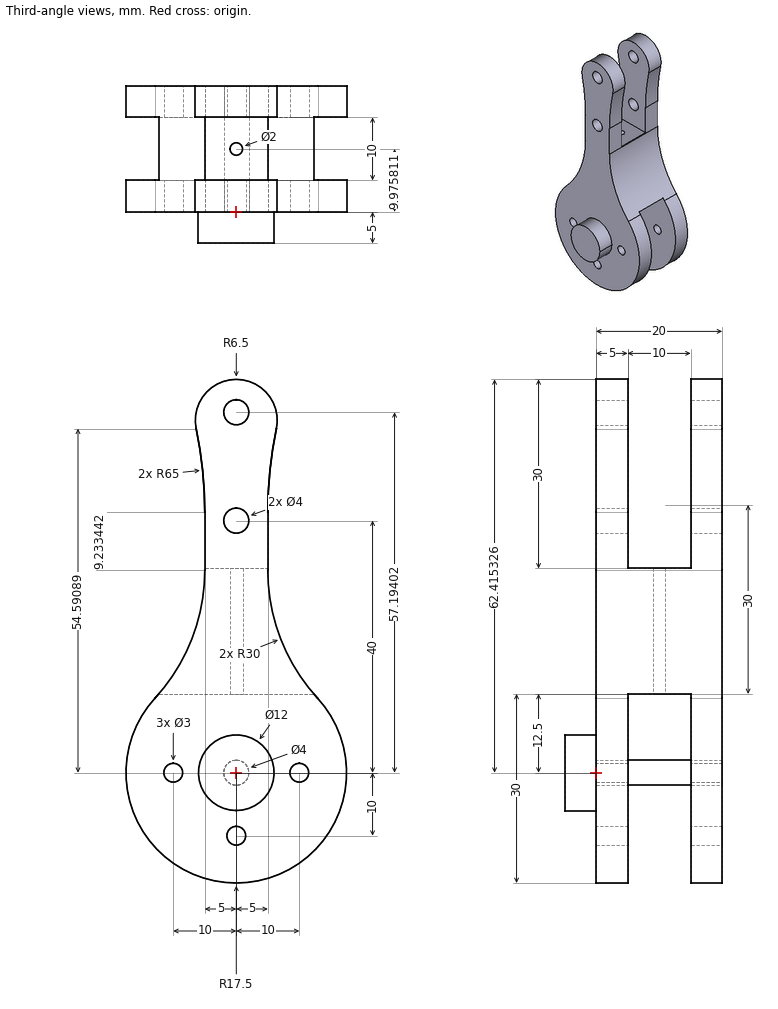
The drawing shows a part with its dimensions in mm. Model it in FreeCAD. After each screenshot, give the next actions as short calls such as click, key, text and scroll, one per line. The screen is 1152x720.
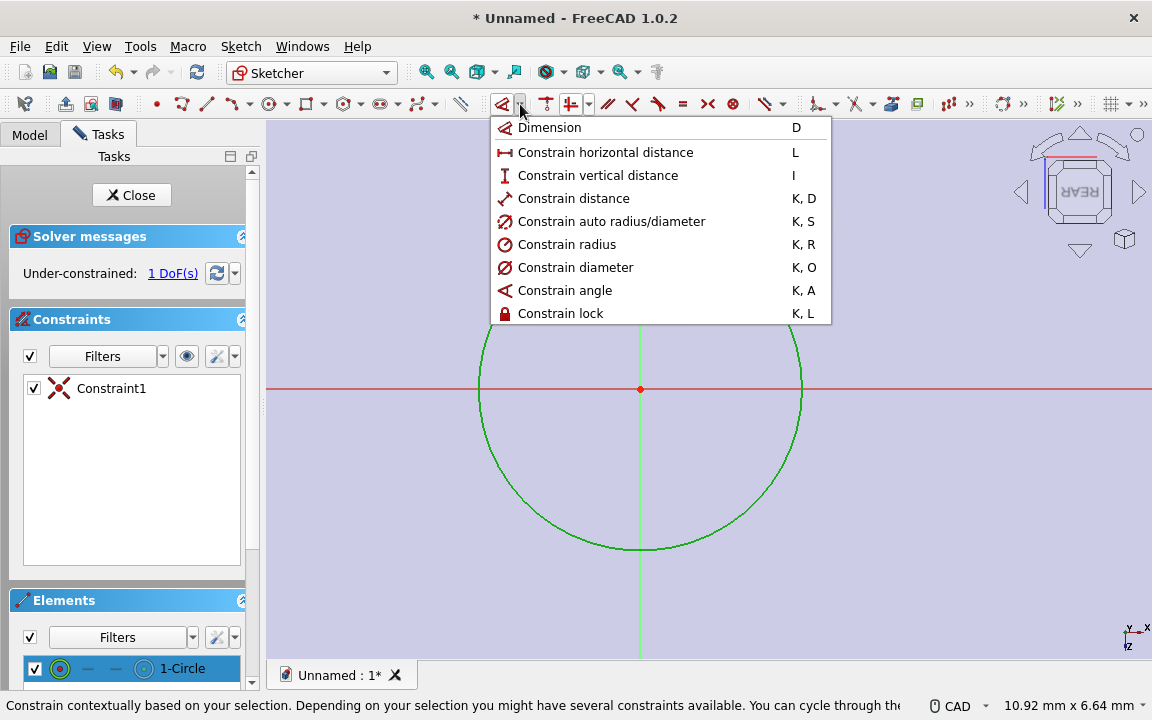
click(661, 268)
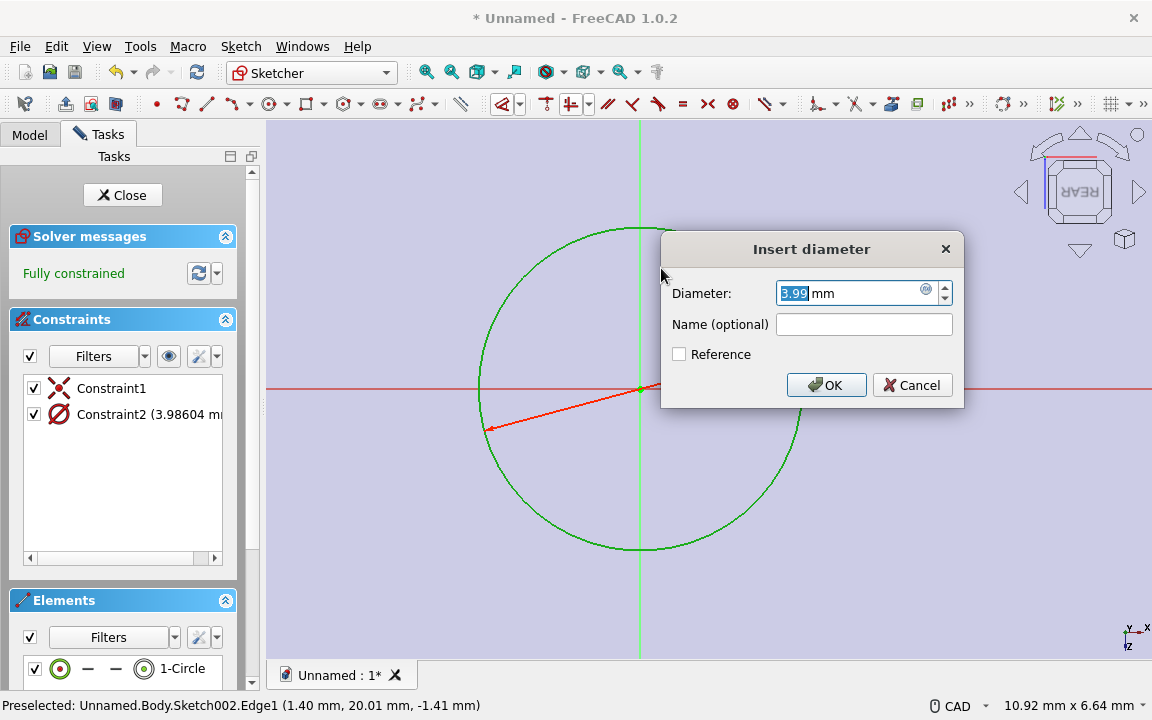
text(4)
key(Return)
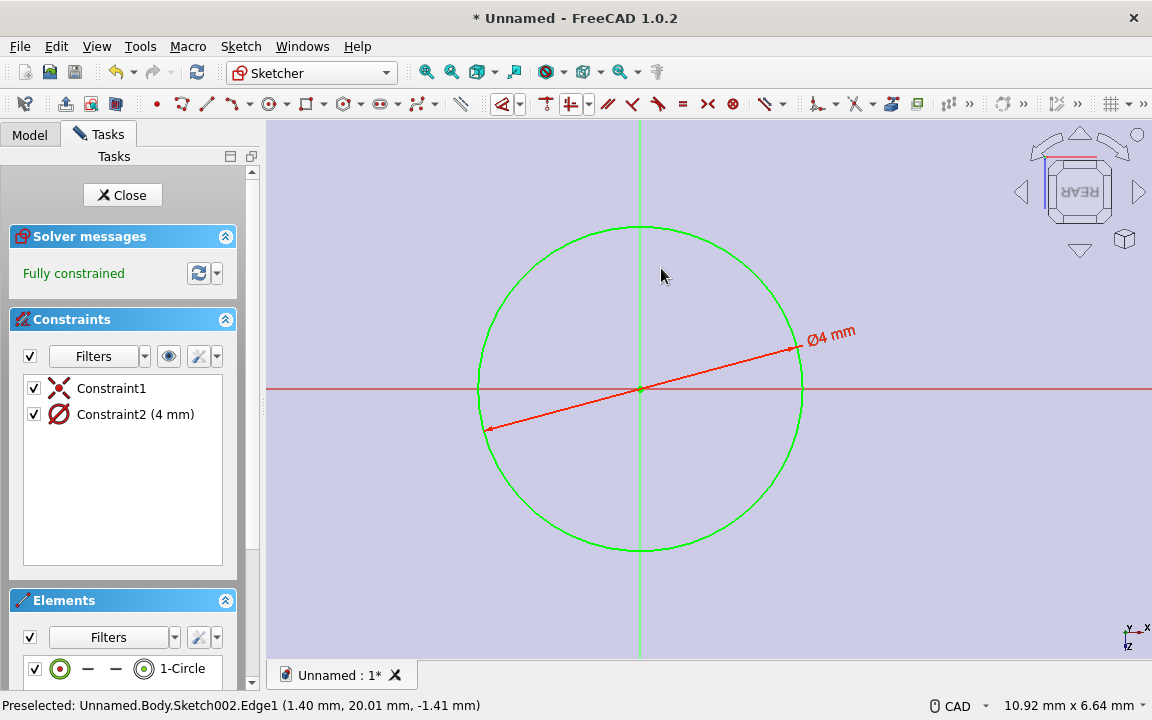
click(123, 195)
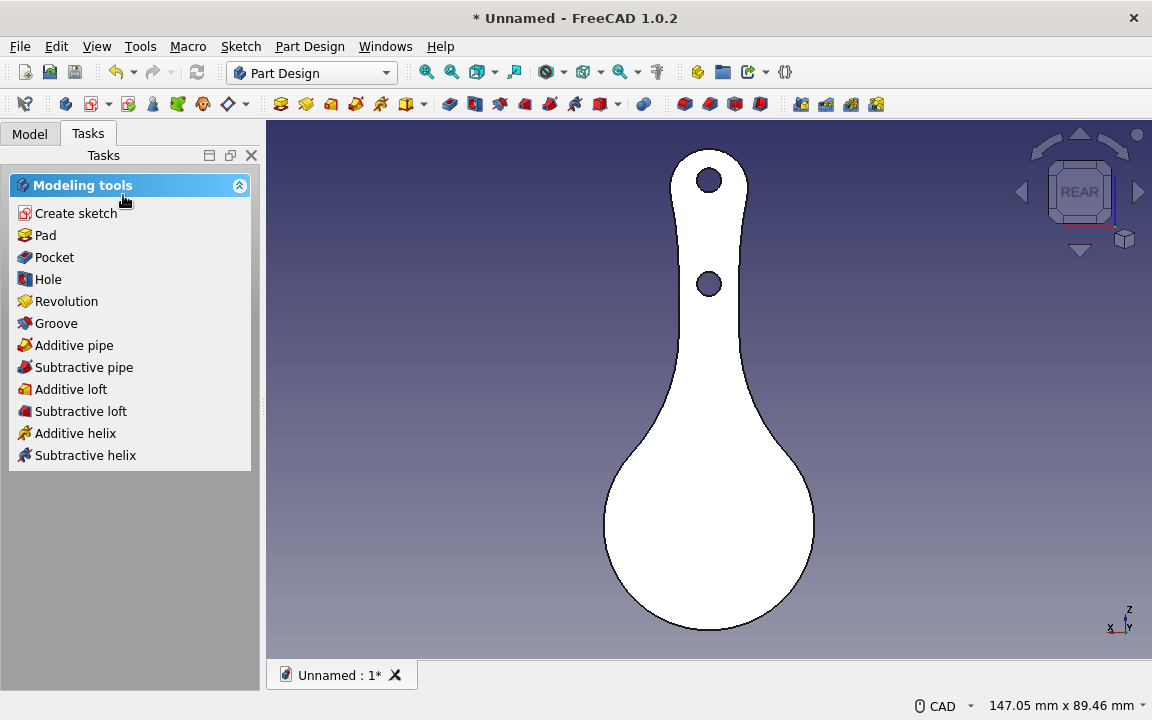
click(450, 104)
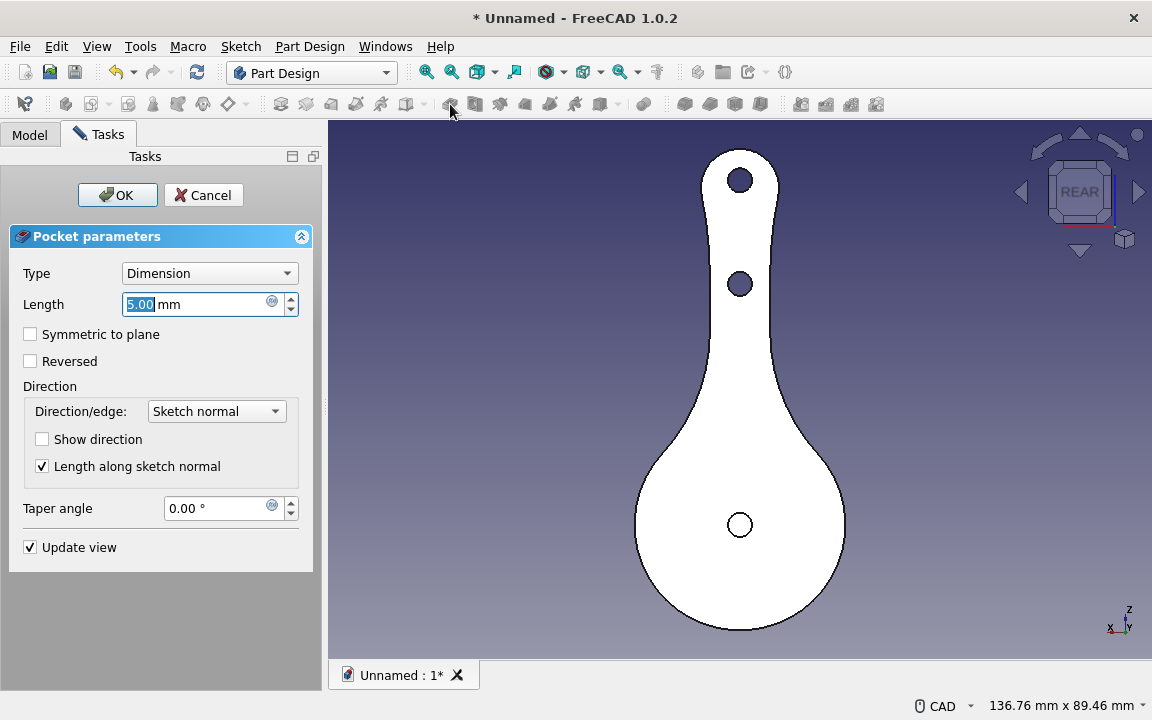
click(210, 274)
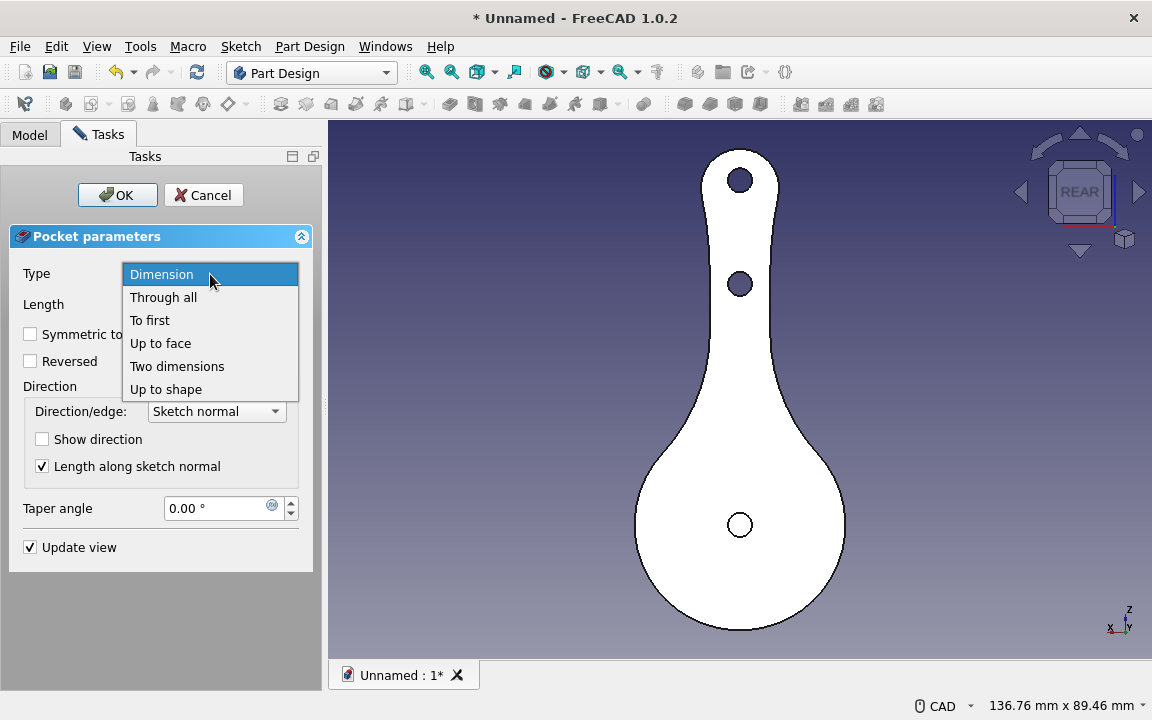
click(208, 298)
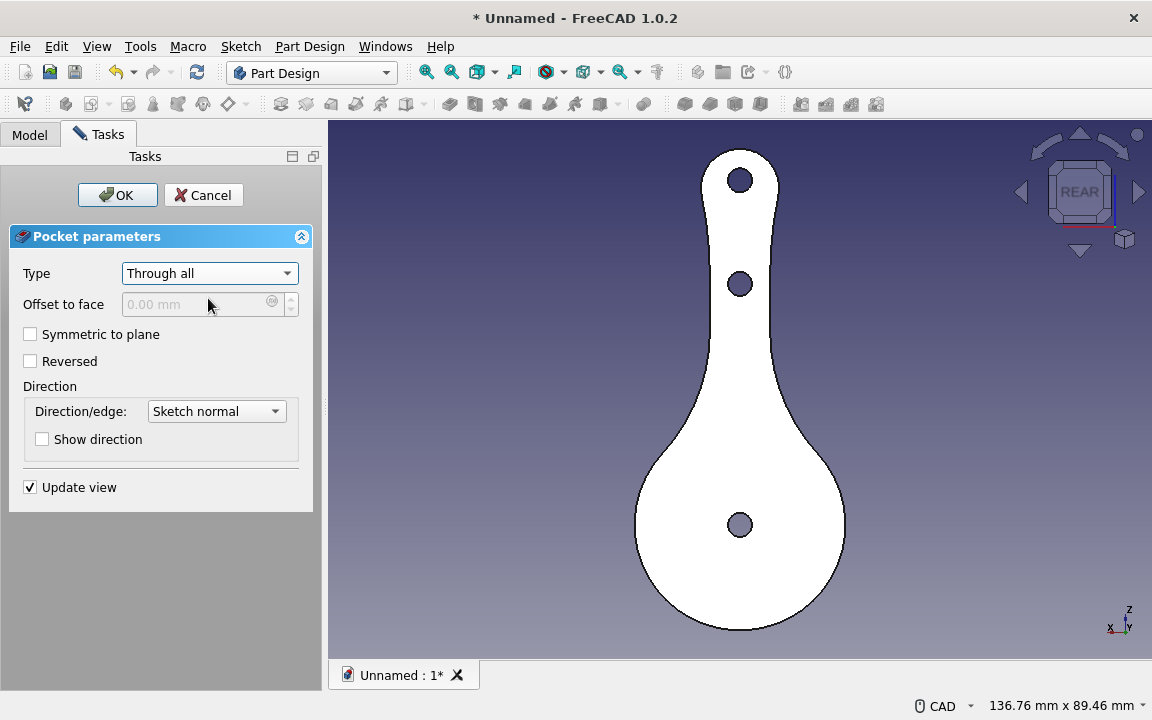
click(118, 195)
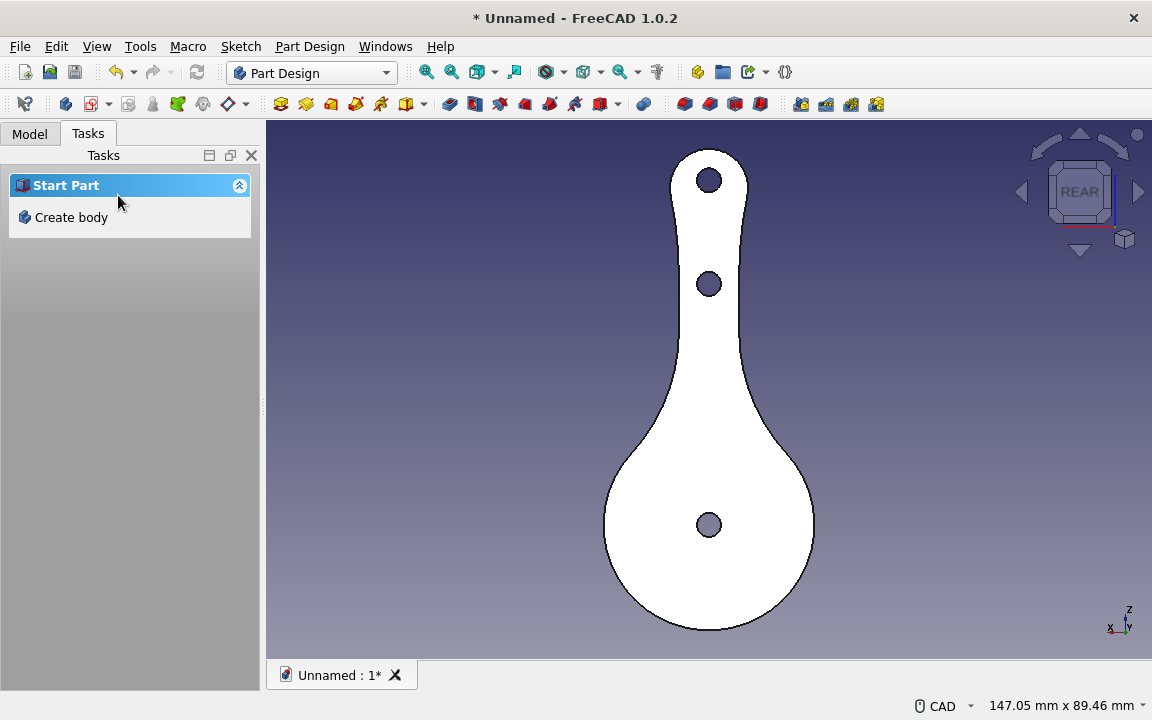
click(709, 457)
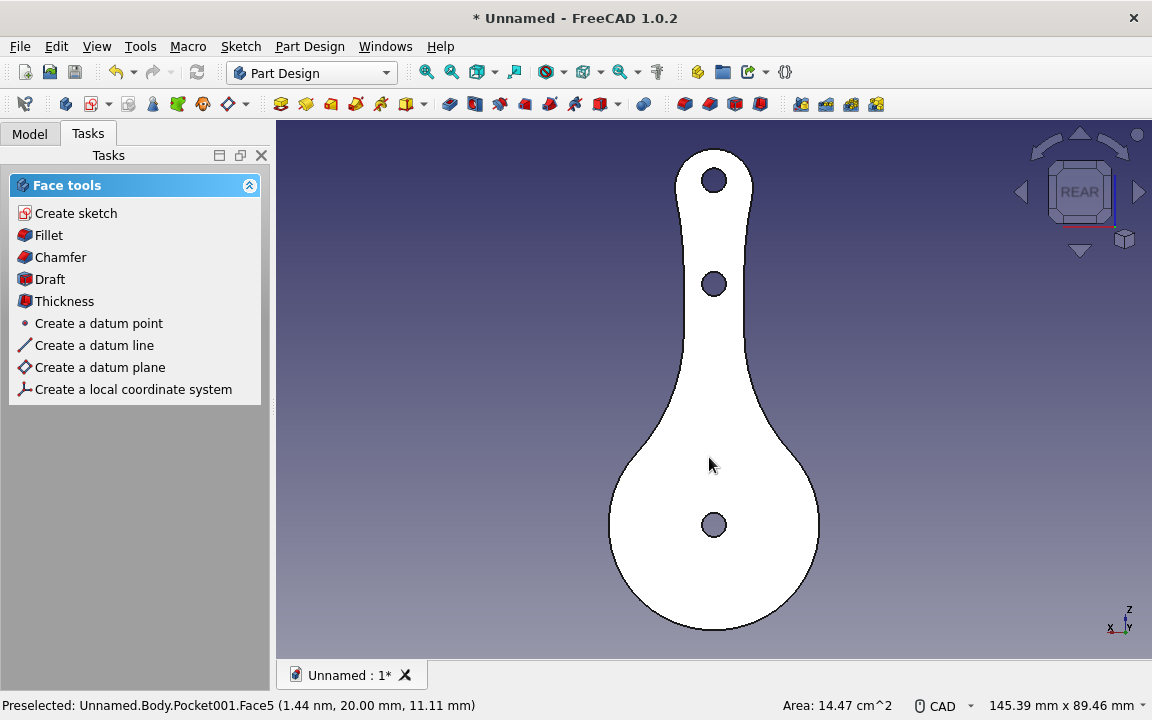
click(90, 104)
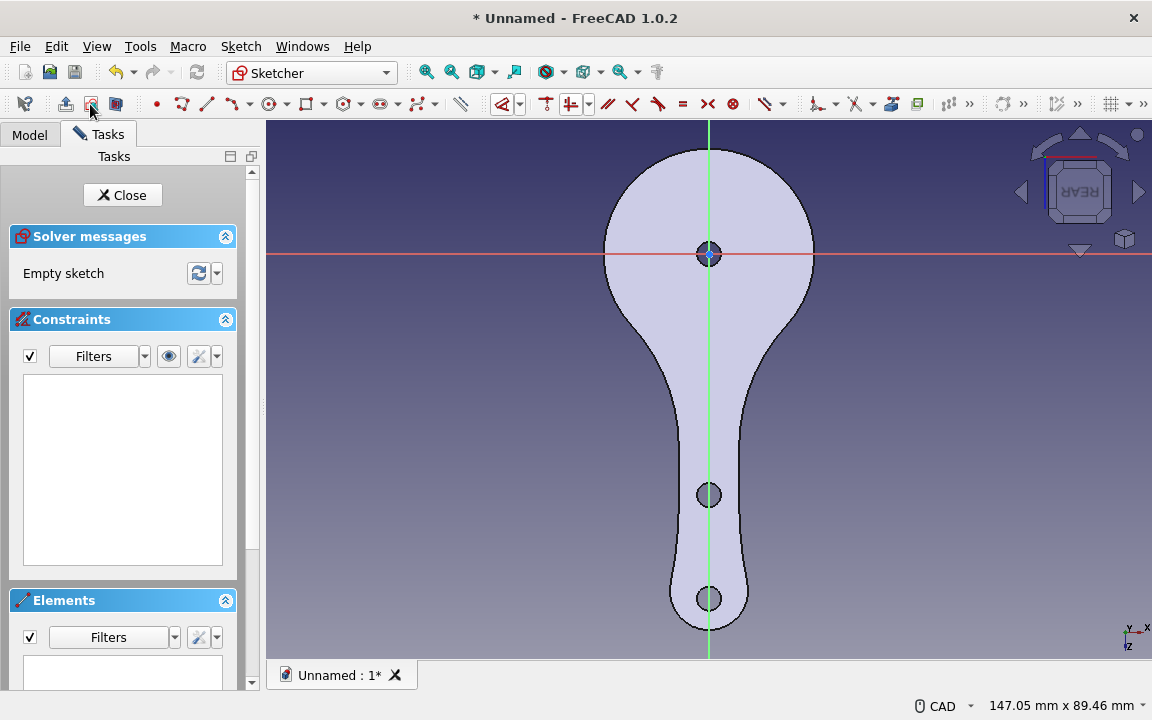
scroll(739, 153, up, 6)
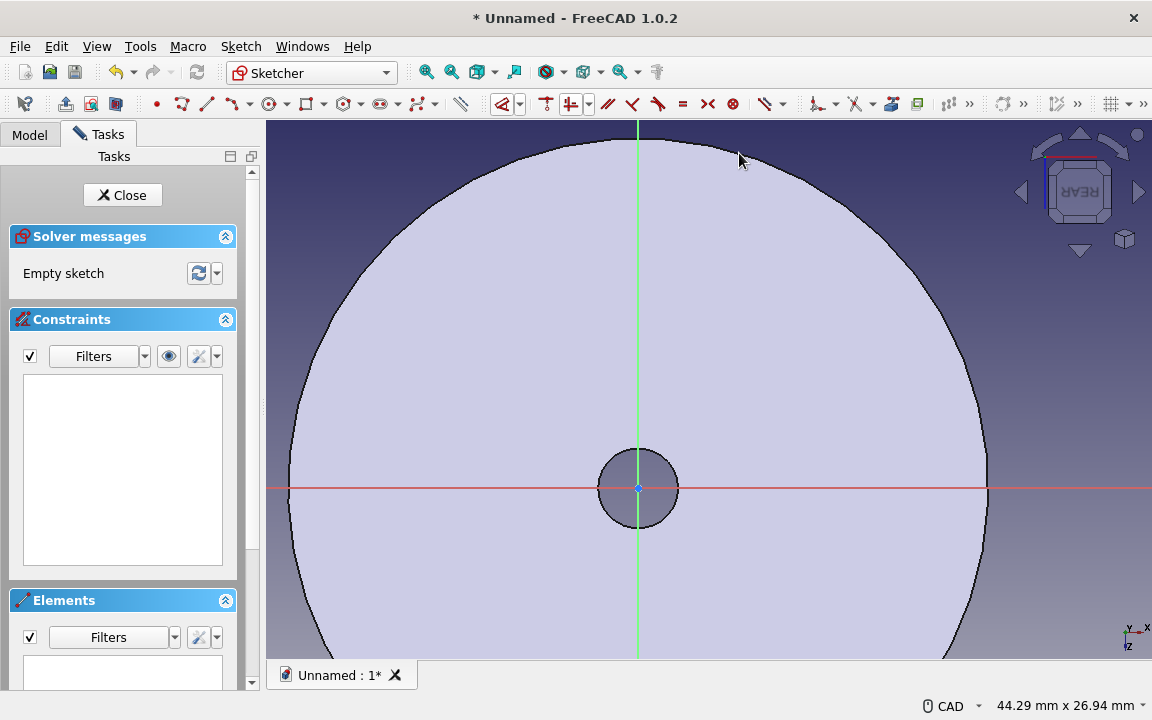
click(268, 104)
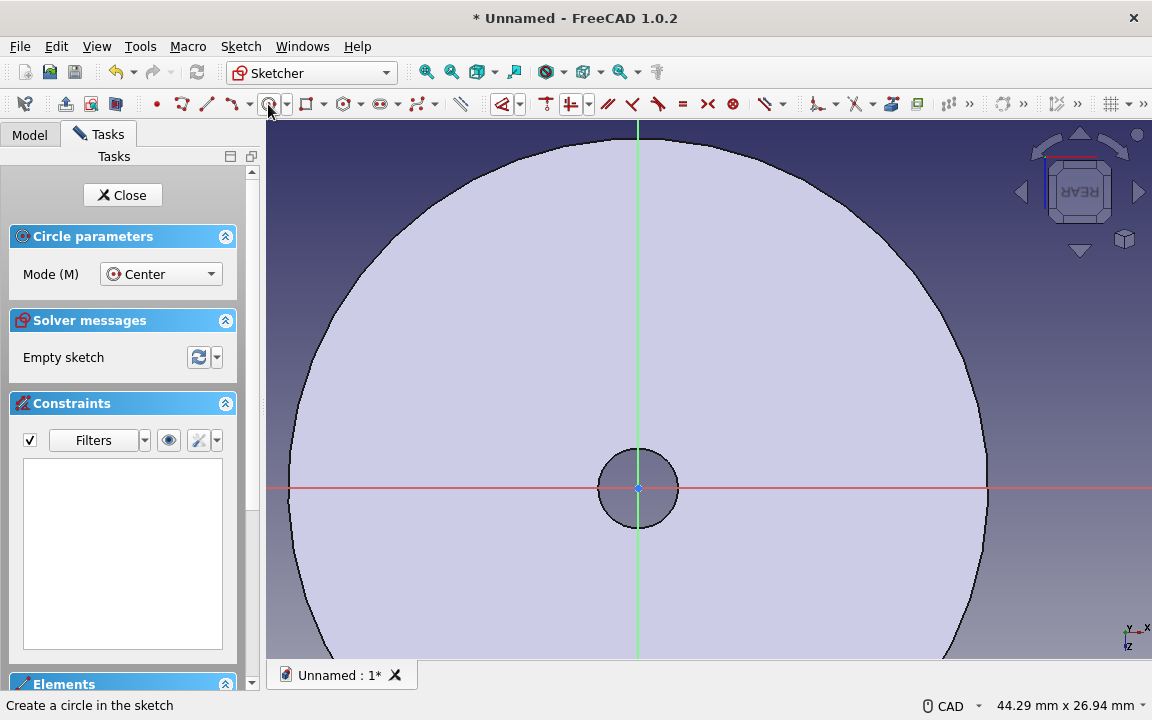
click(438, 488)
click(459, 467)